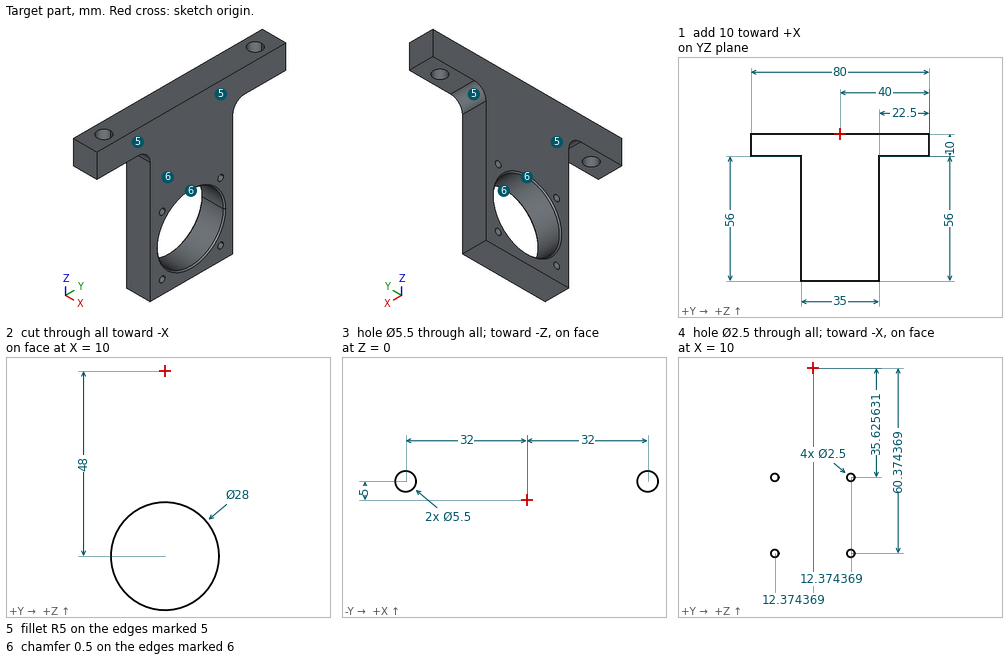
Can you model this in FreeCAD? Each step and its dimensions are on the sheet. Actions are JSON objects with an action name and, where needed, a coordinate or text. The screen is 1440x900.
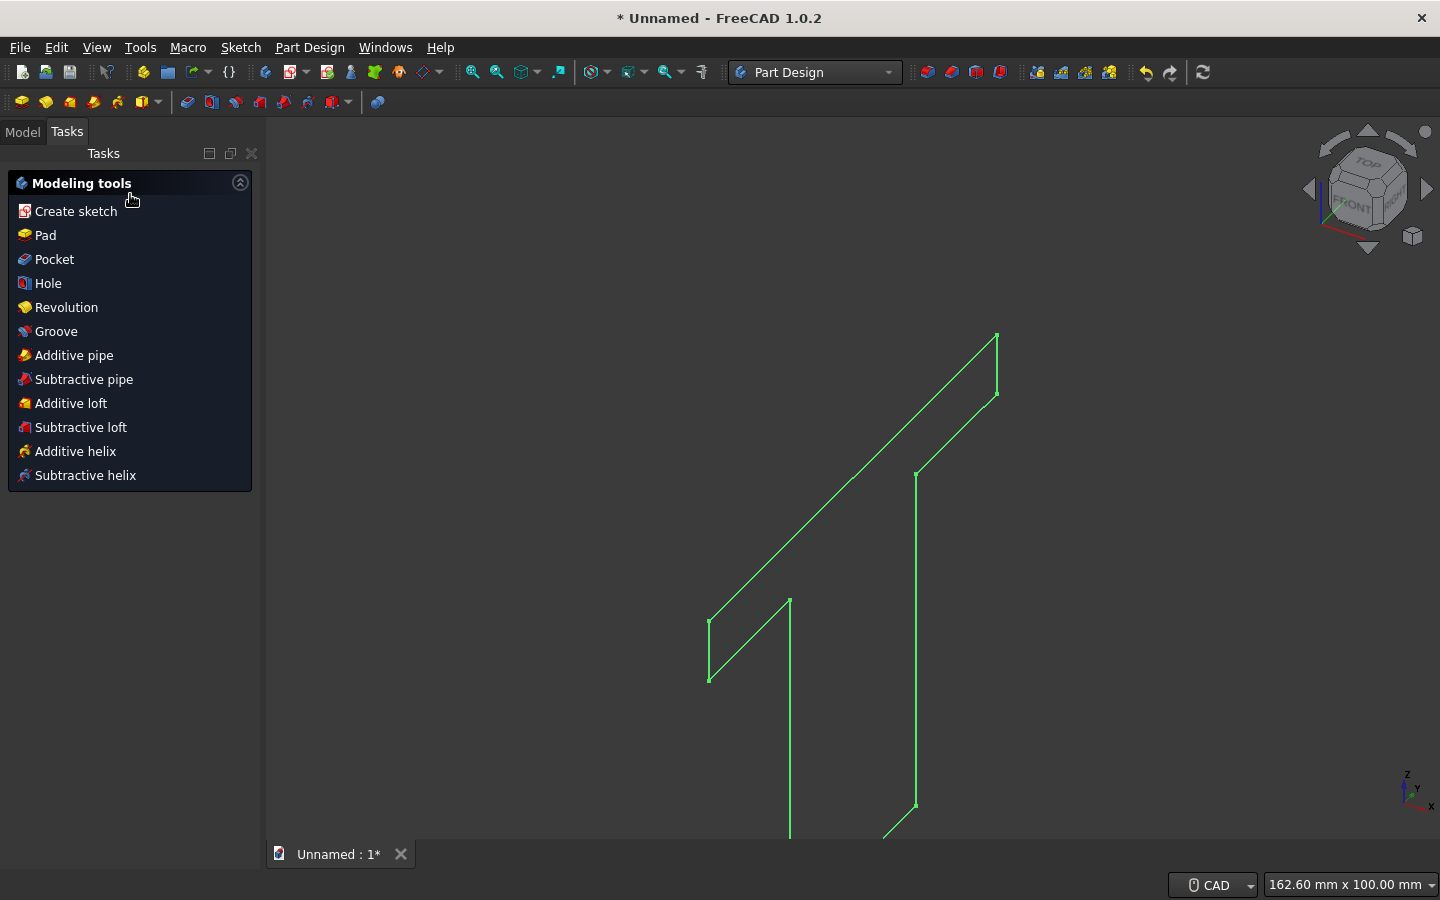
{"action": "left_click", "coordinate": [22, 102]}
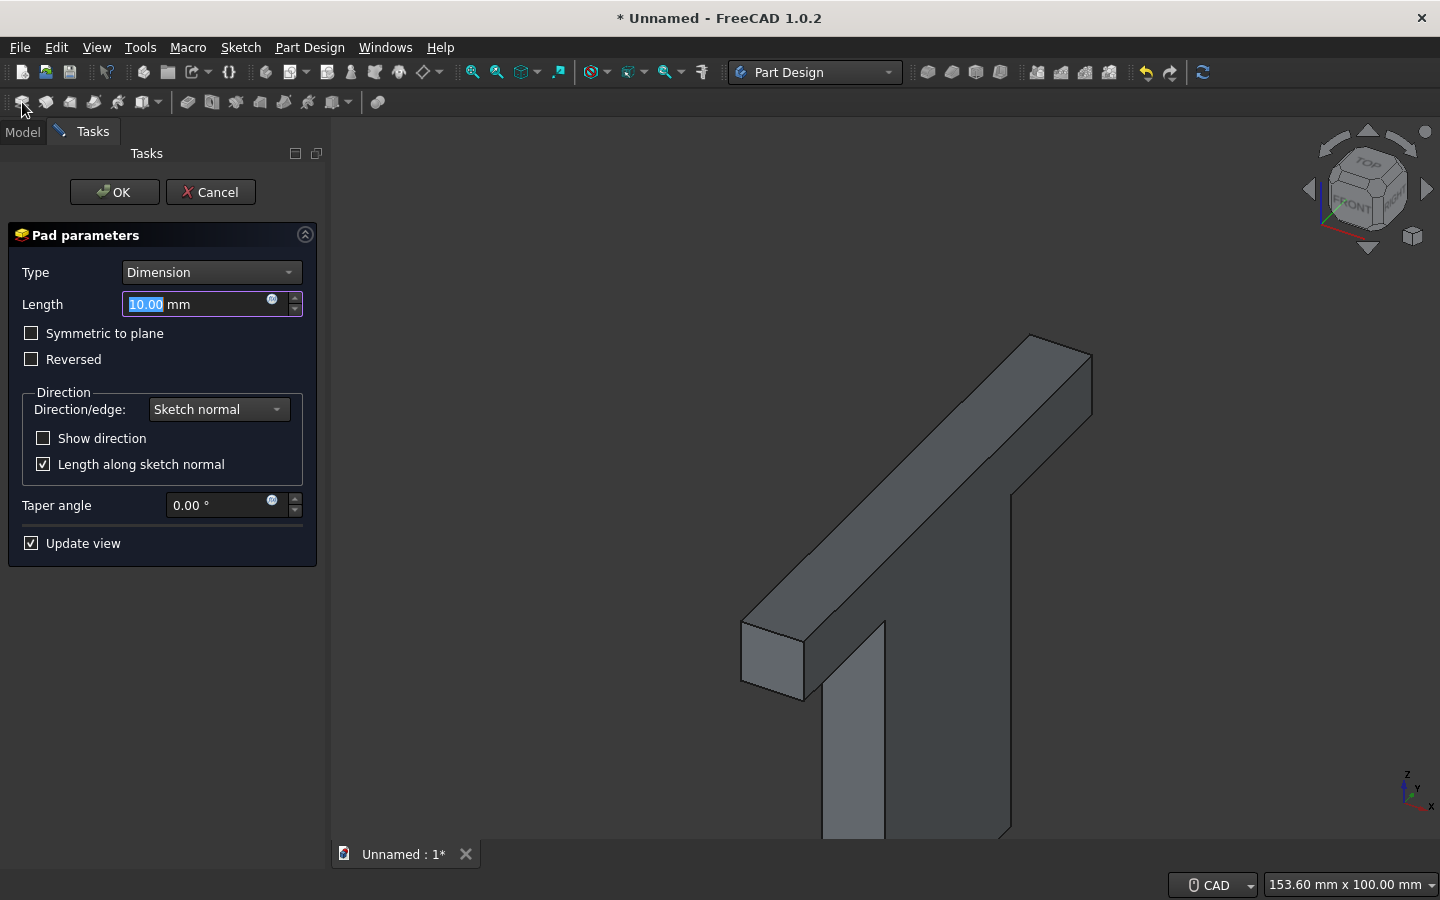
{"action": "type", "text": "10"}
{"action": "key", "text": "Tab"}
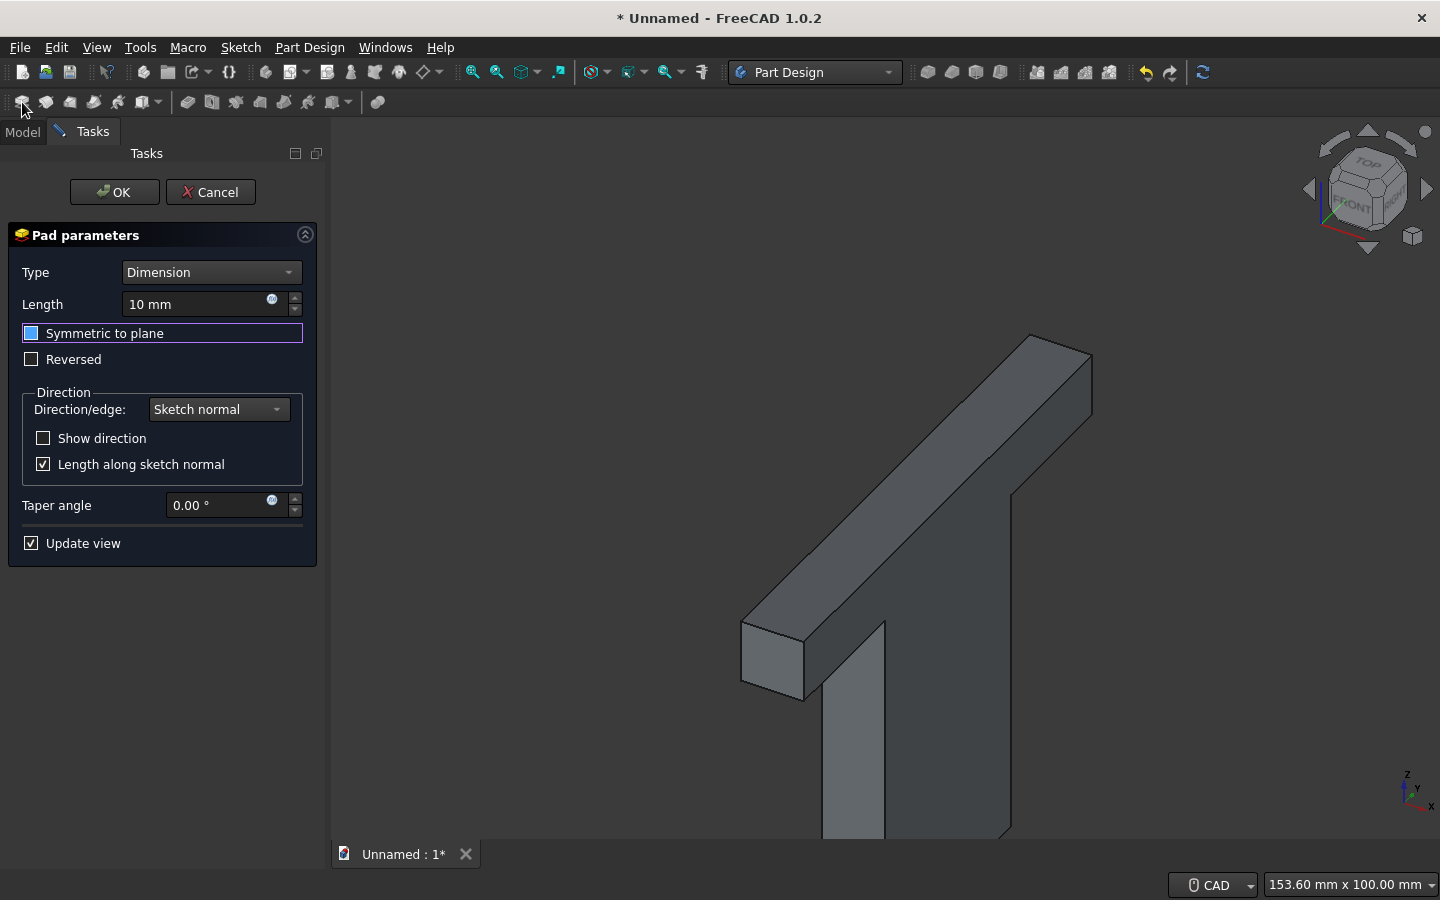
{"action": "left_click", "coordinate": [115, 192]}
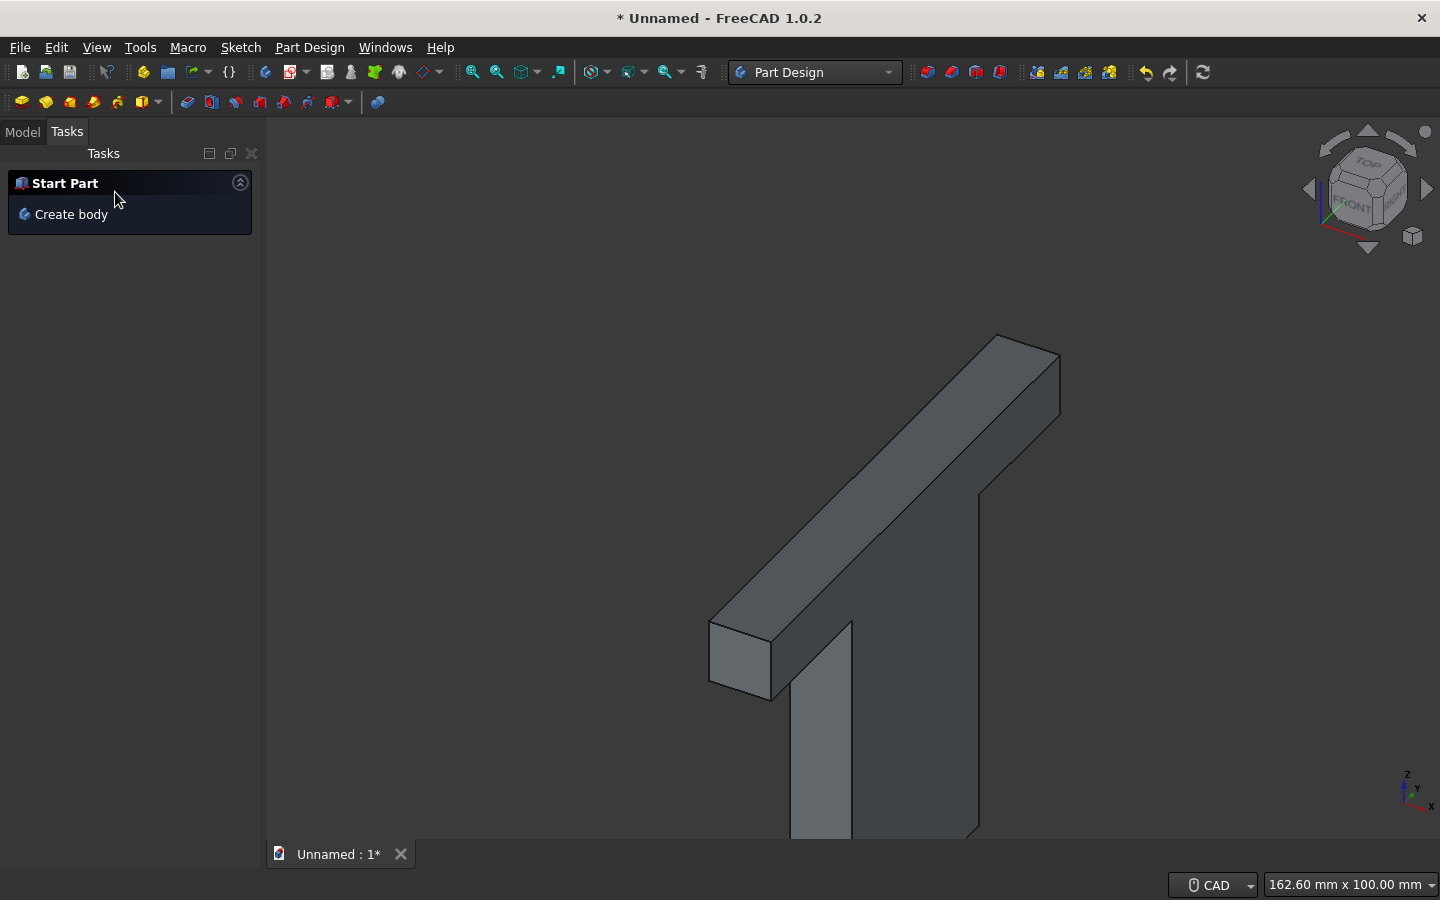
{"action": "left_click", "coordinate": [474, 72]}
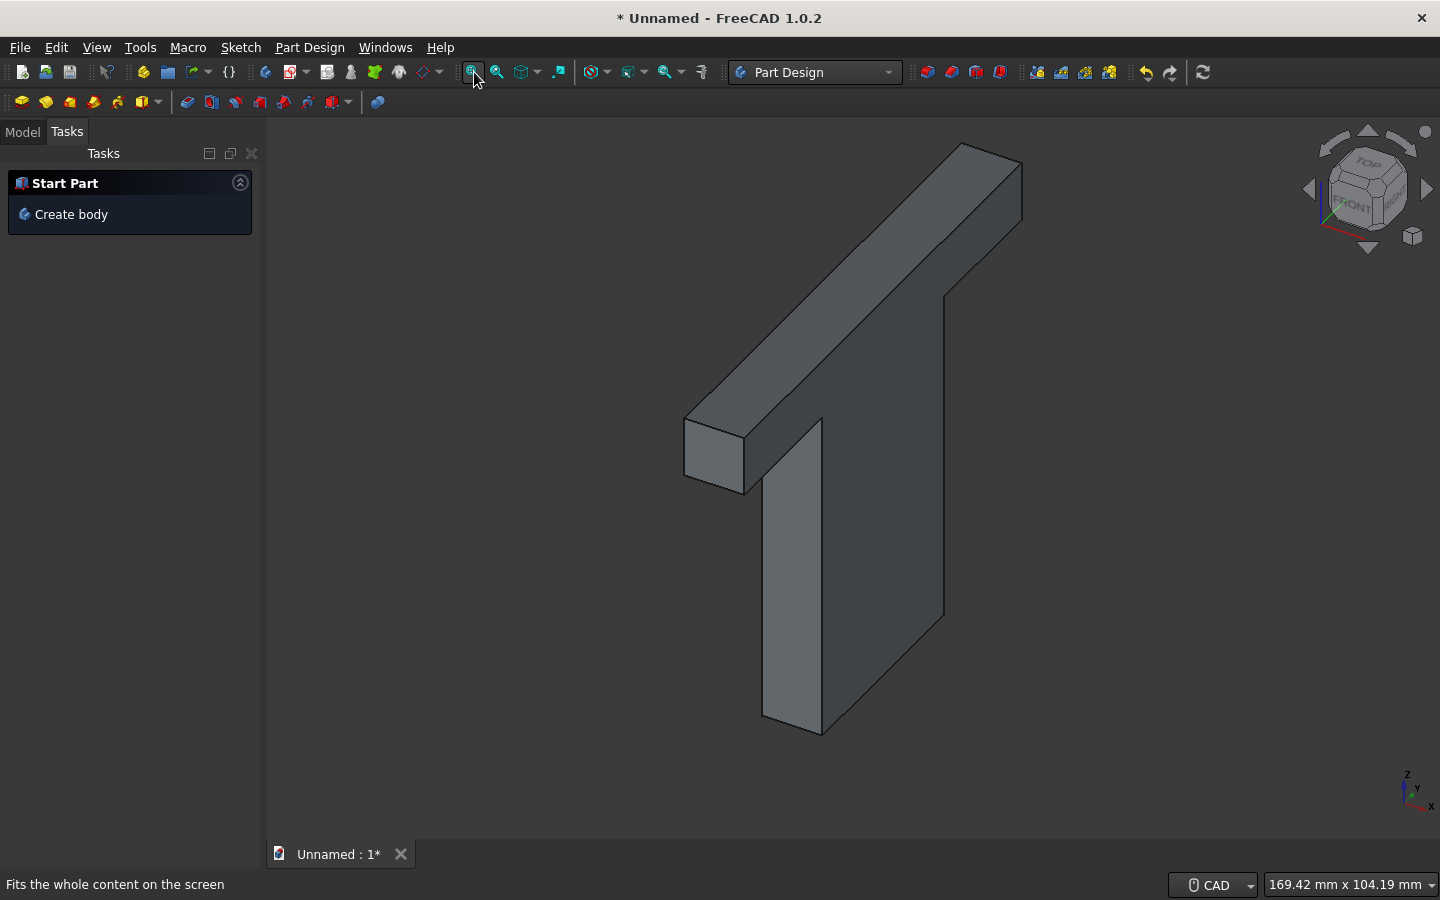
{"action": "left_click", "coordinate": [883, 540]}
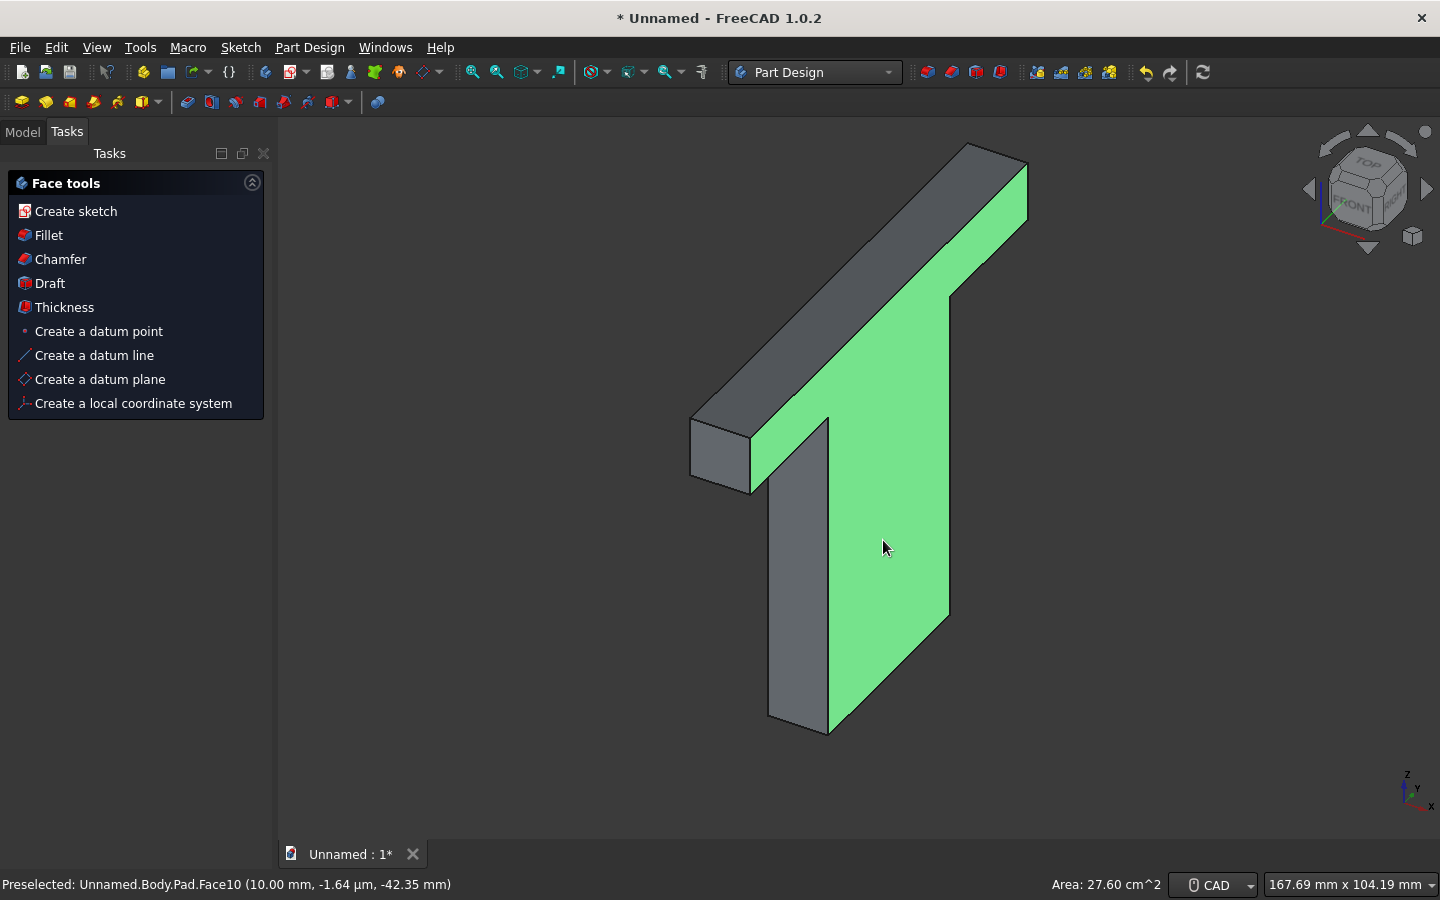
{"action": "left_click", "coordinate": [290, 72]}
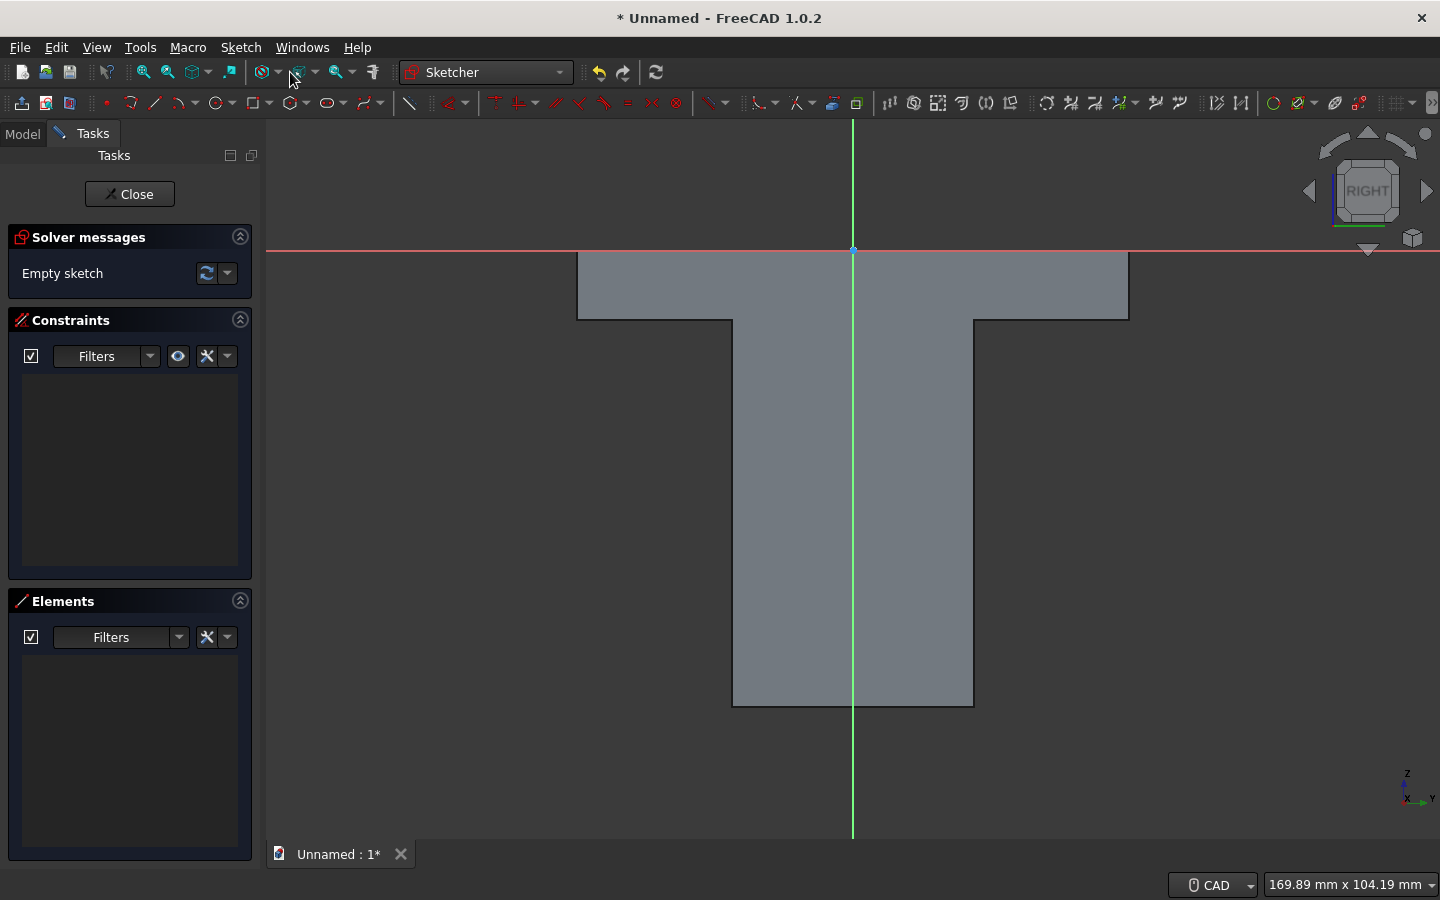
{"action": "left_click", "coordinate": [216, 104]}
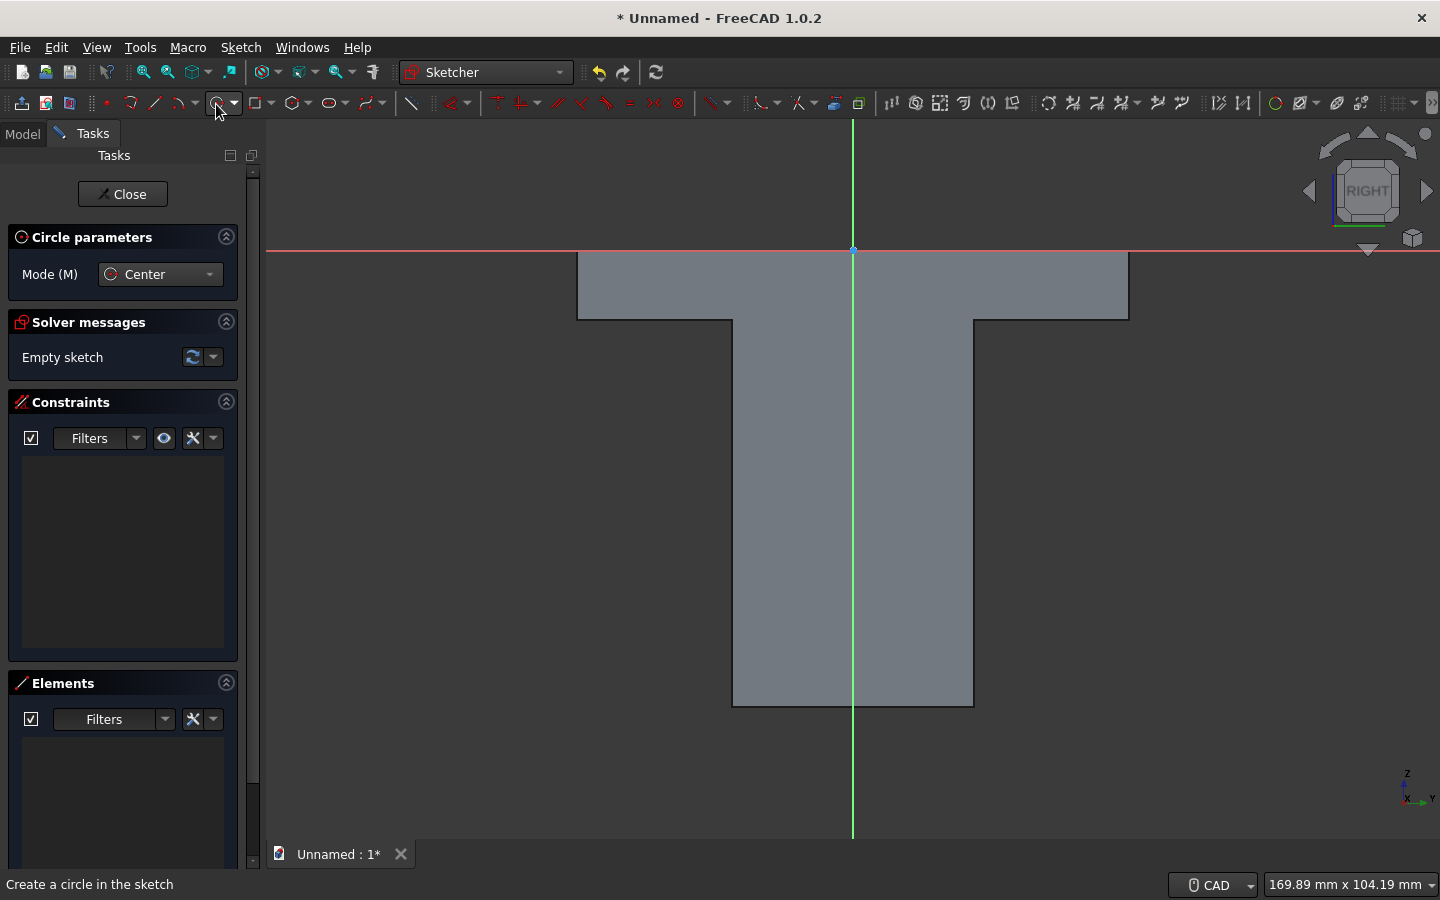
{"action": "left_click", "coordinate": [853, 583]}
{"action": "mouse_move", "coordinate": [921, 514]}